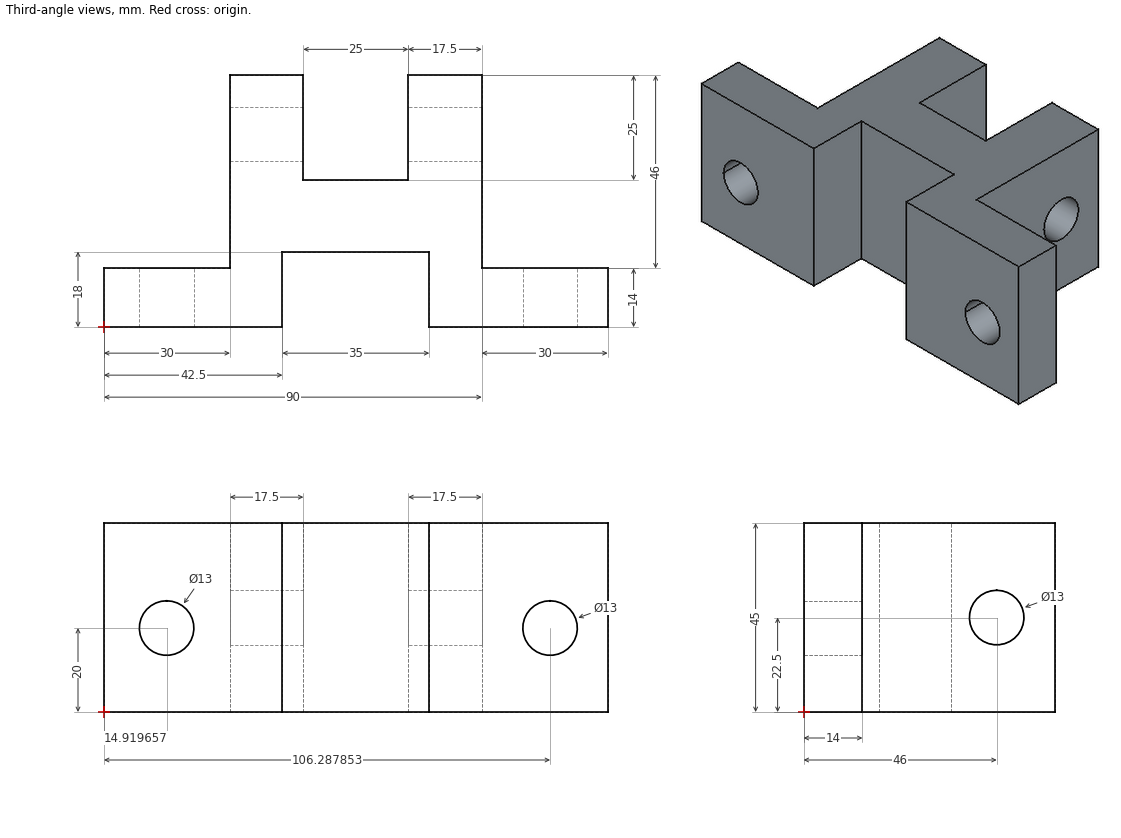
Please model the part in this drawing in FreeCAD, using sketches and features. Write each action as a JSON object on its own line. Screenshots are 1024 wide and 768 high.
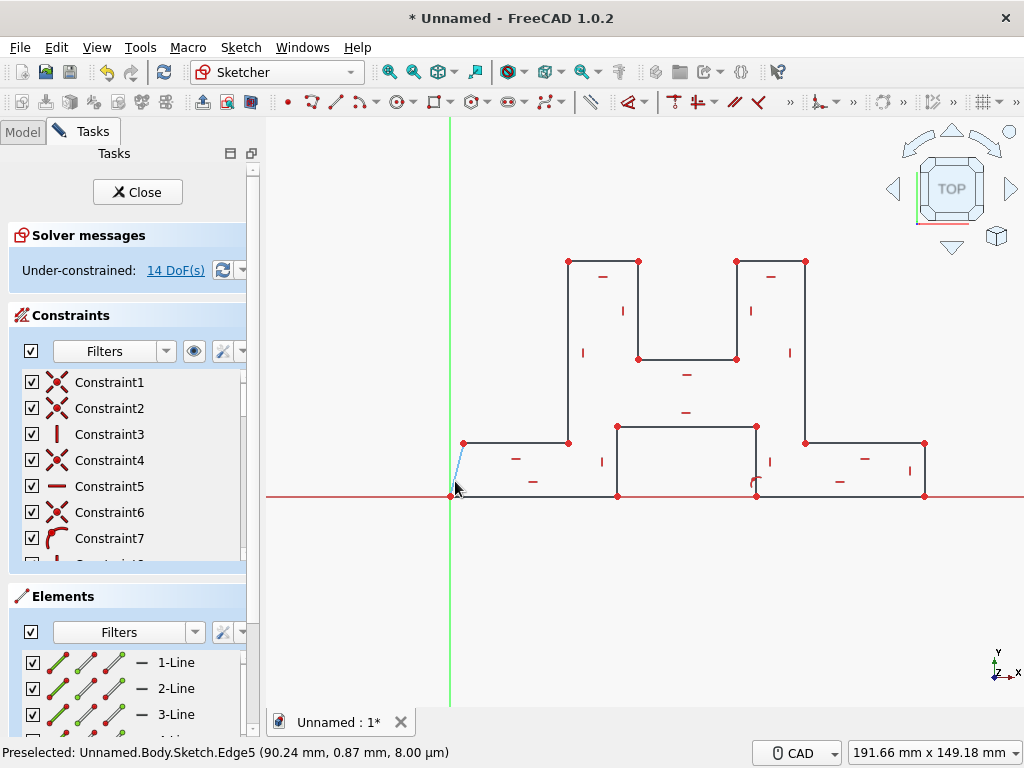
{"action": "left_click", "coordinate": [454, 481]}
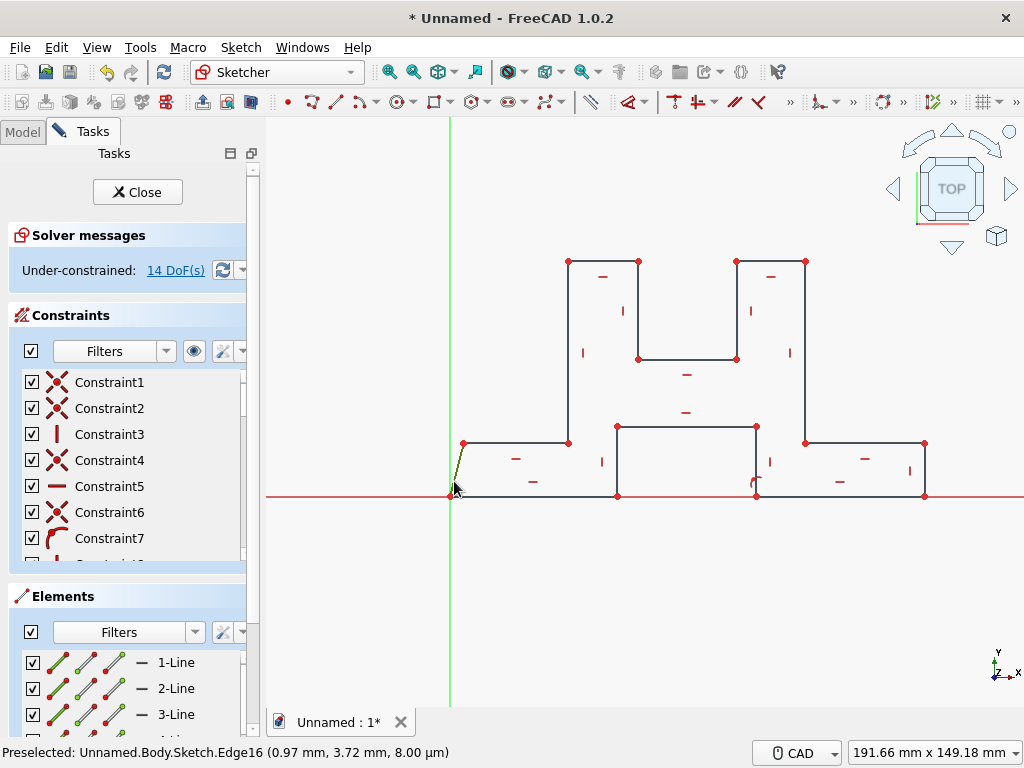
{"action": "left_click", "coordinate": [716, 102]}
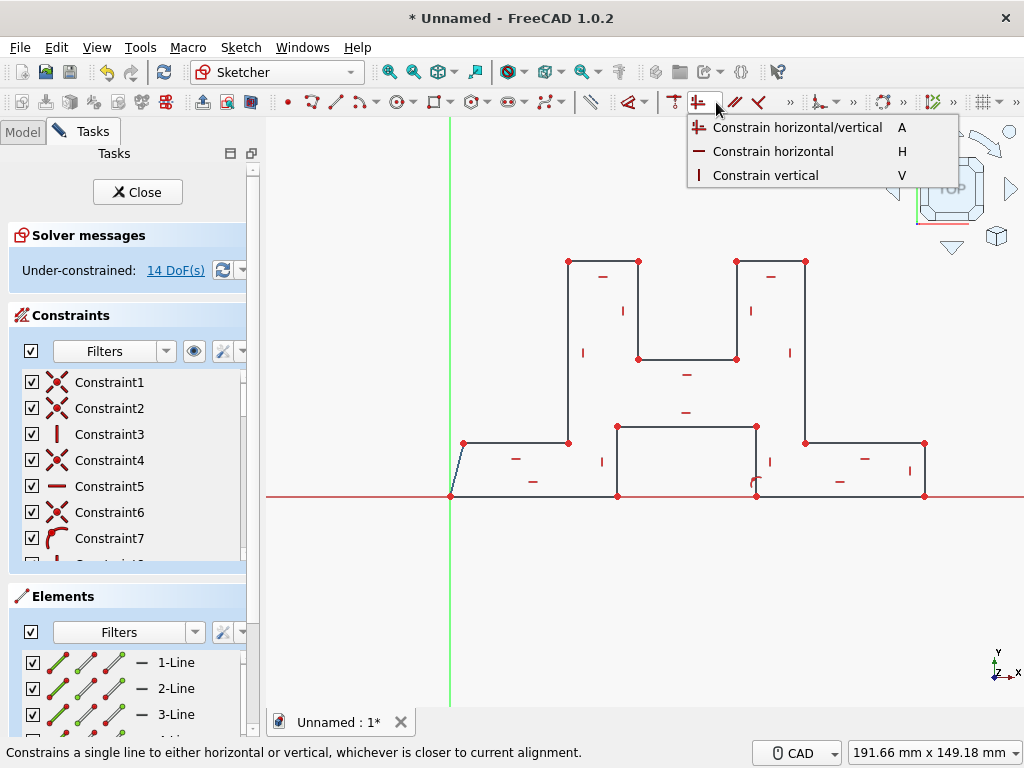
{"action": "left_click", "coordinate": [823, 175]}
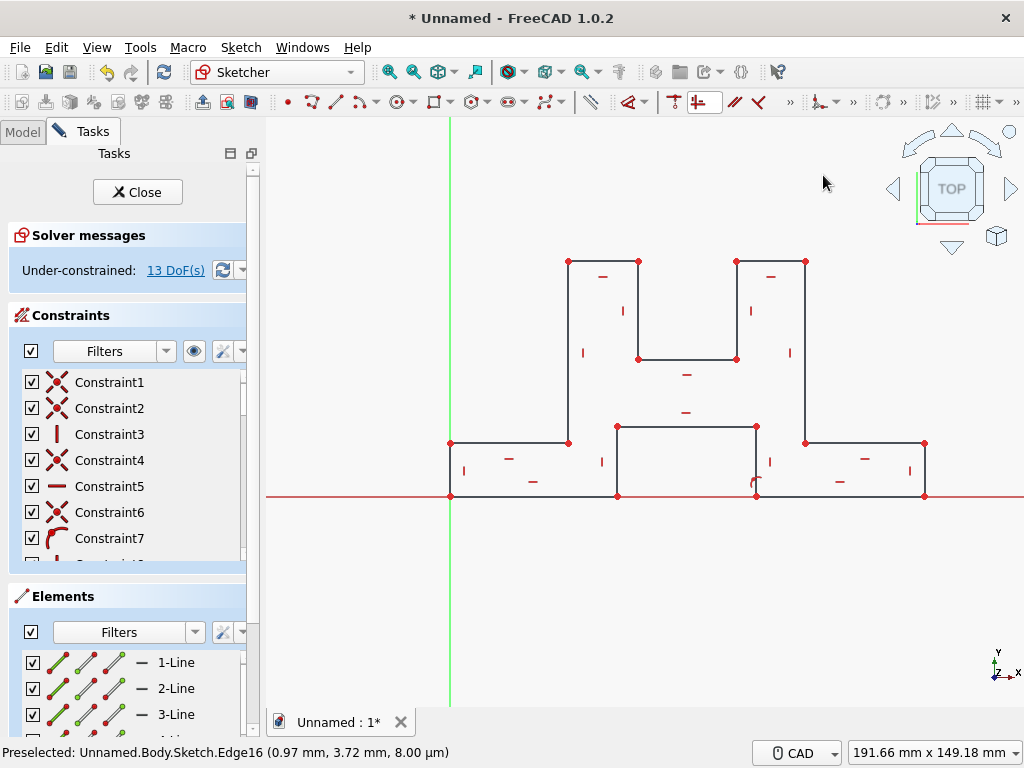
{"action": "left_click", "coordinate": [617, 476]}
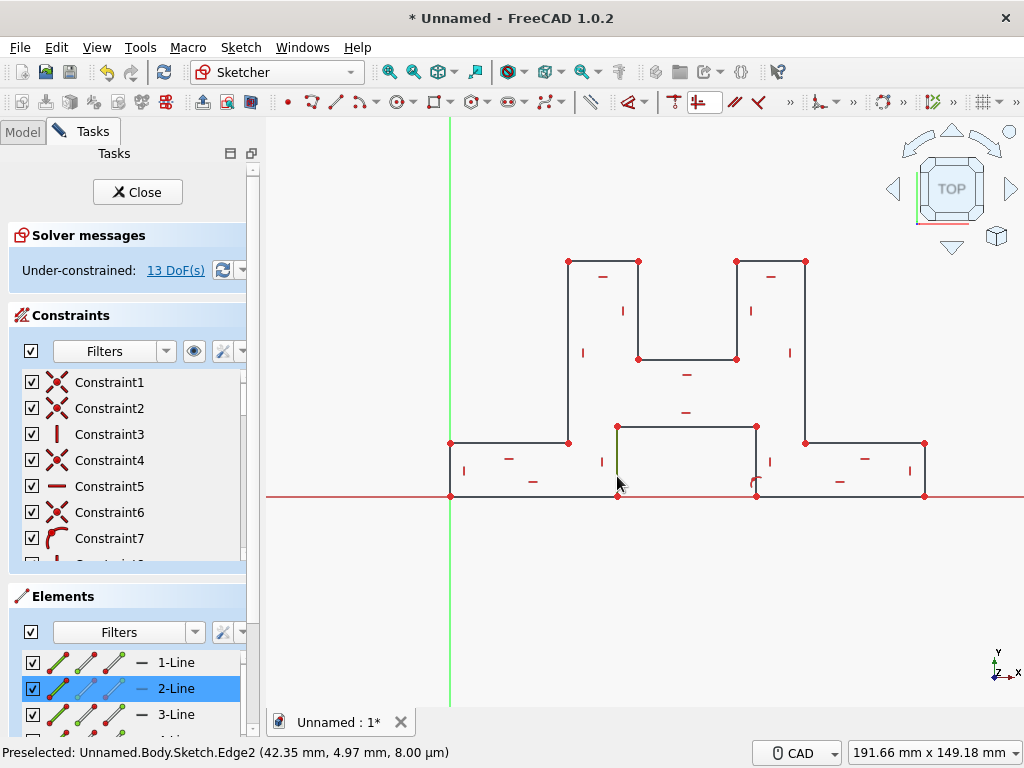
{"action": "key", "text": "i"}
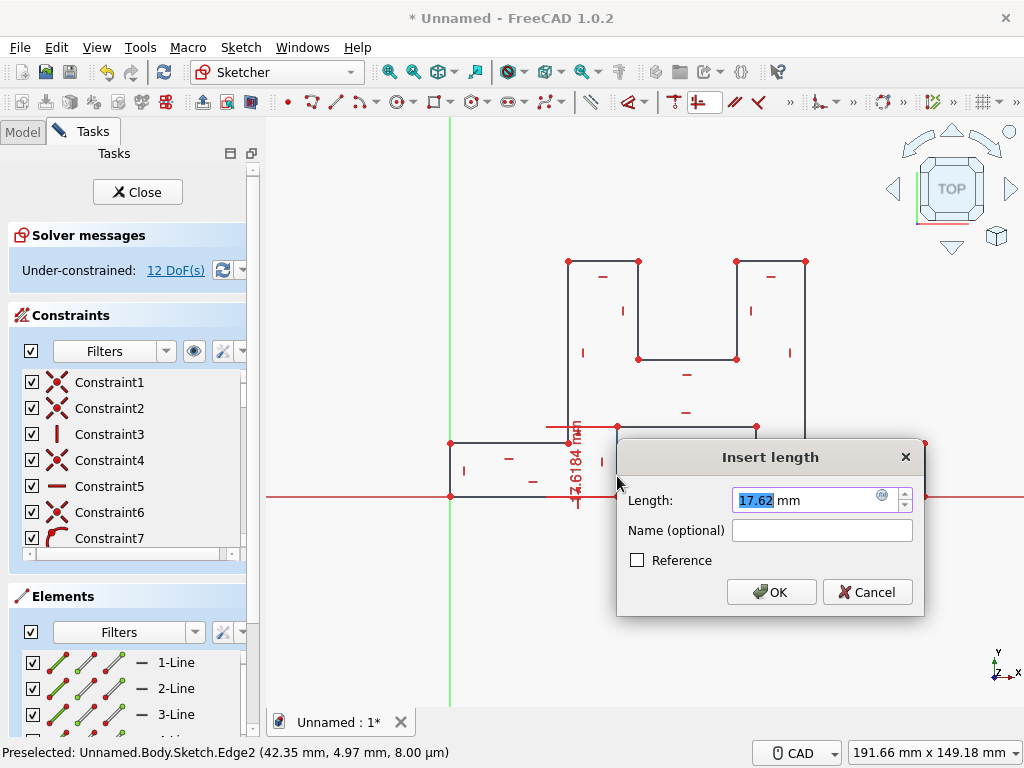
{"action": "type", "text": "18"}
{"action": "key", "text": "Return"}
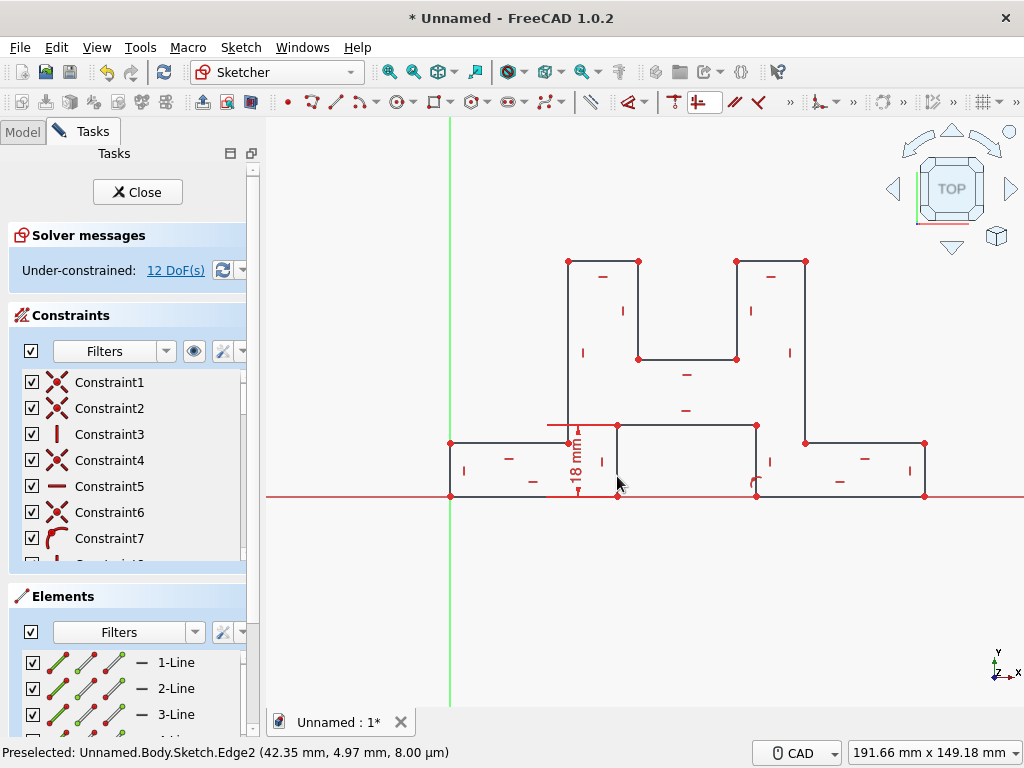
{"action": "left_click", "coordinate": [659, 425]}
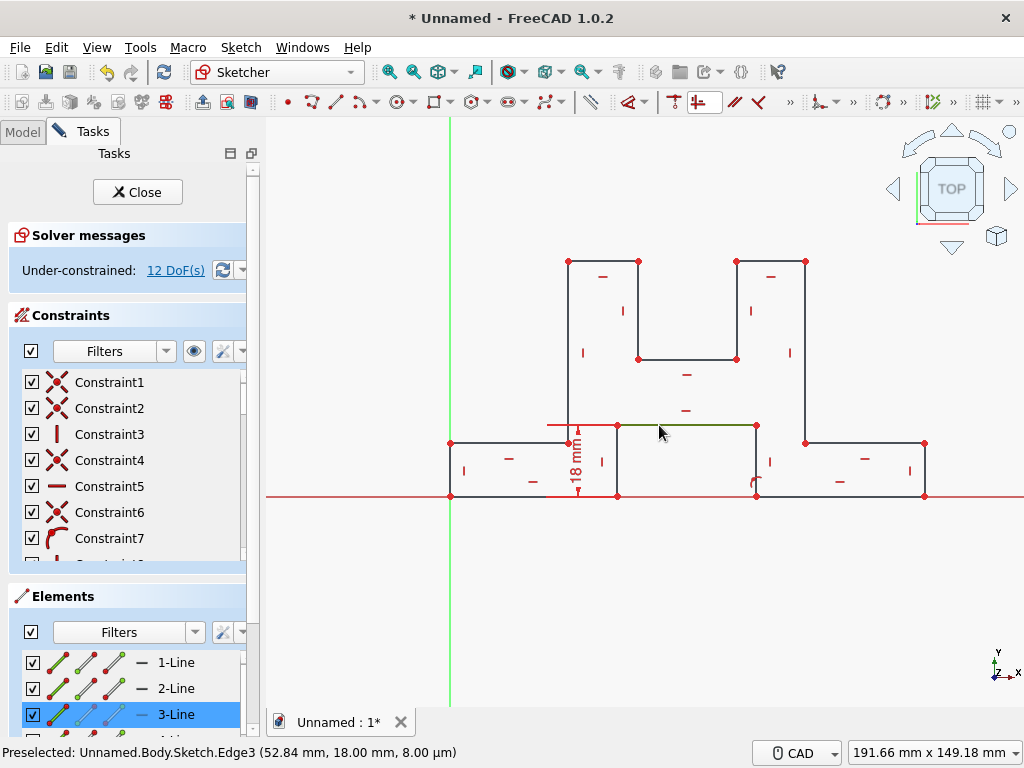
{"action": "key", "text": "l"}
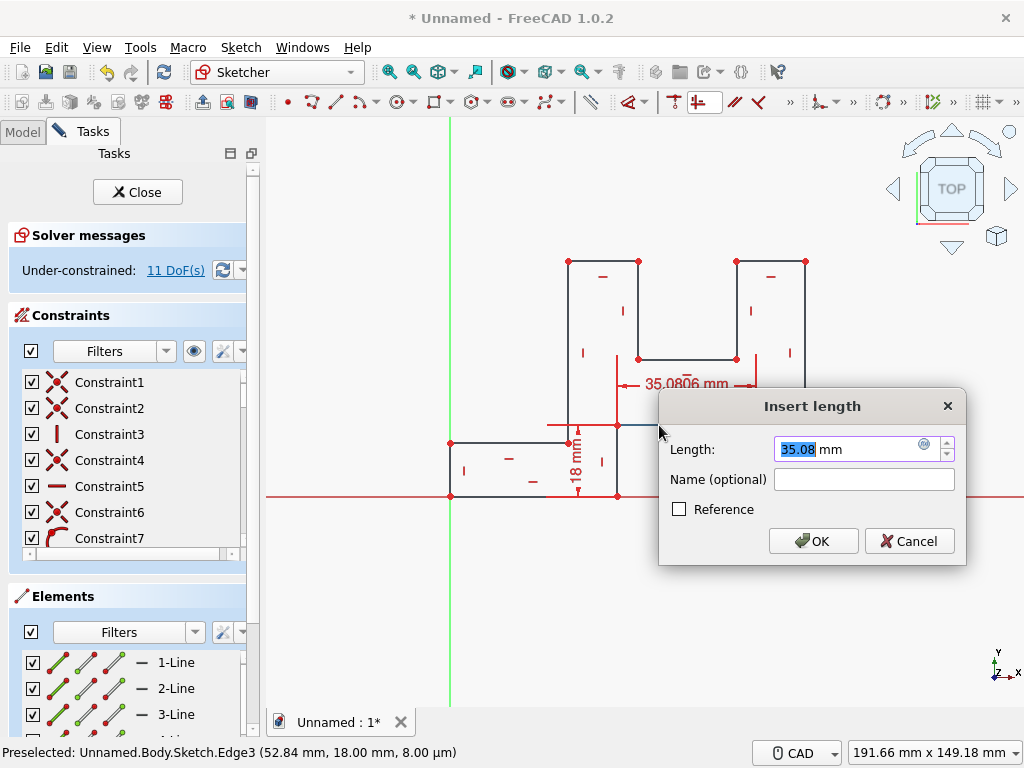
{"action": "type", "text": "35"}
{"action": "key", "text": "Return"}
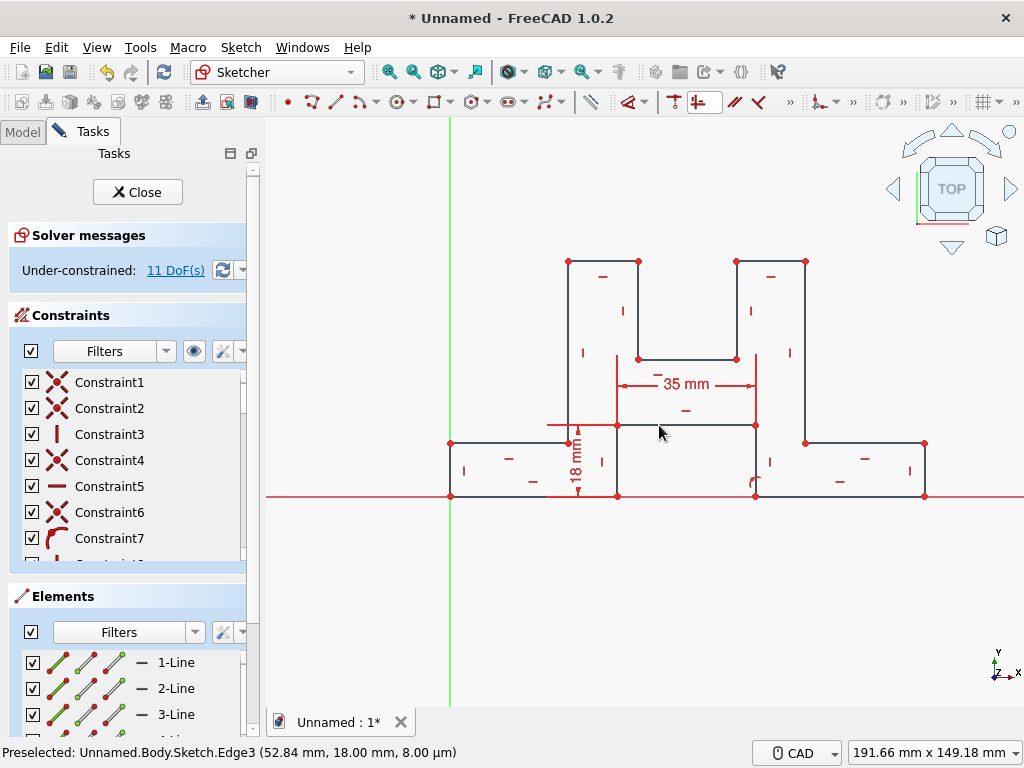
{"action": "scroll", "coordinate": [294, 565], "scroll_direction": "down", "scroll_amount": 1}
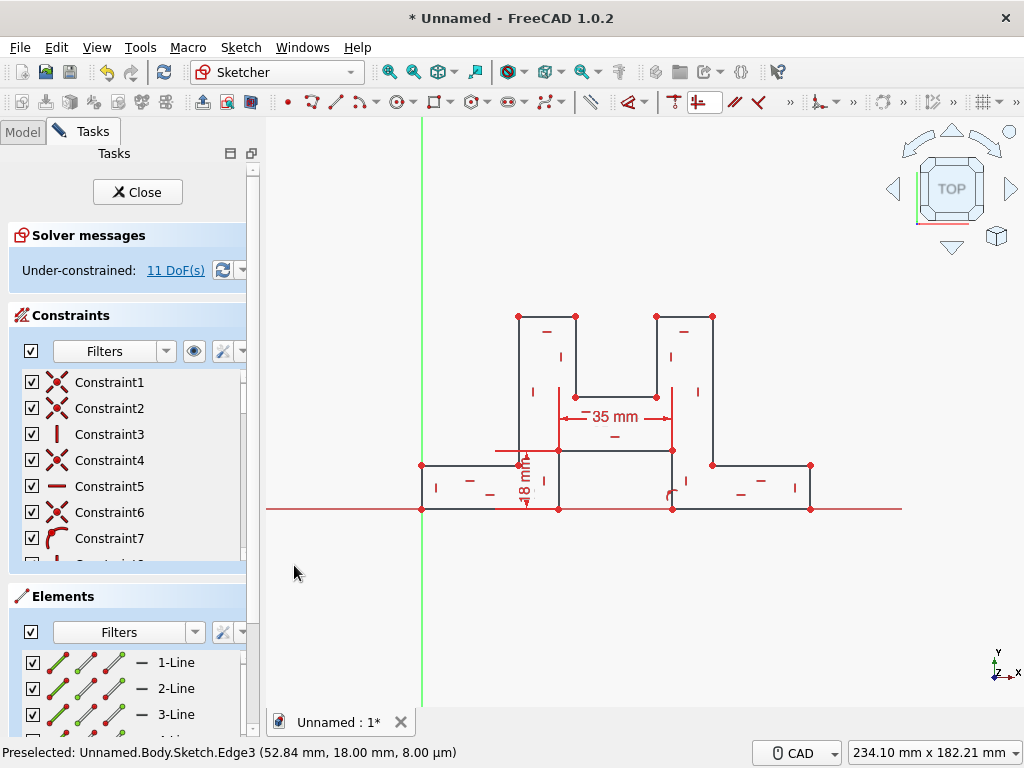
{"action": "left_click", "coordinate": [810, 496]}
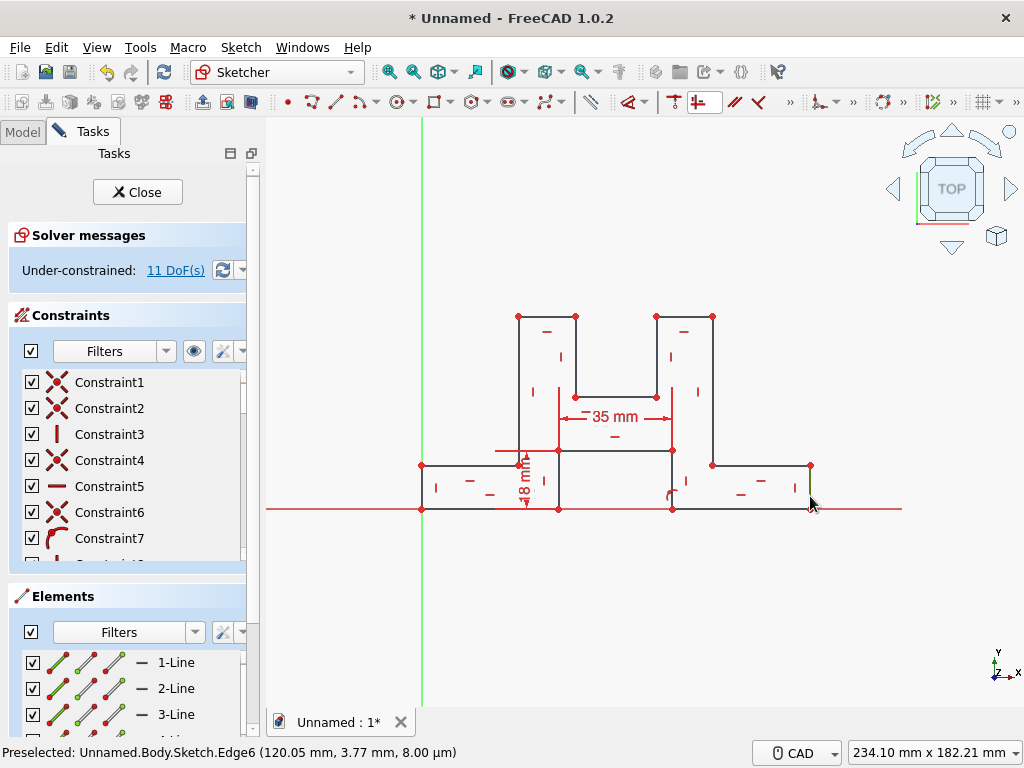
{"action": "key", "text": "i"}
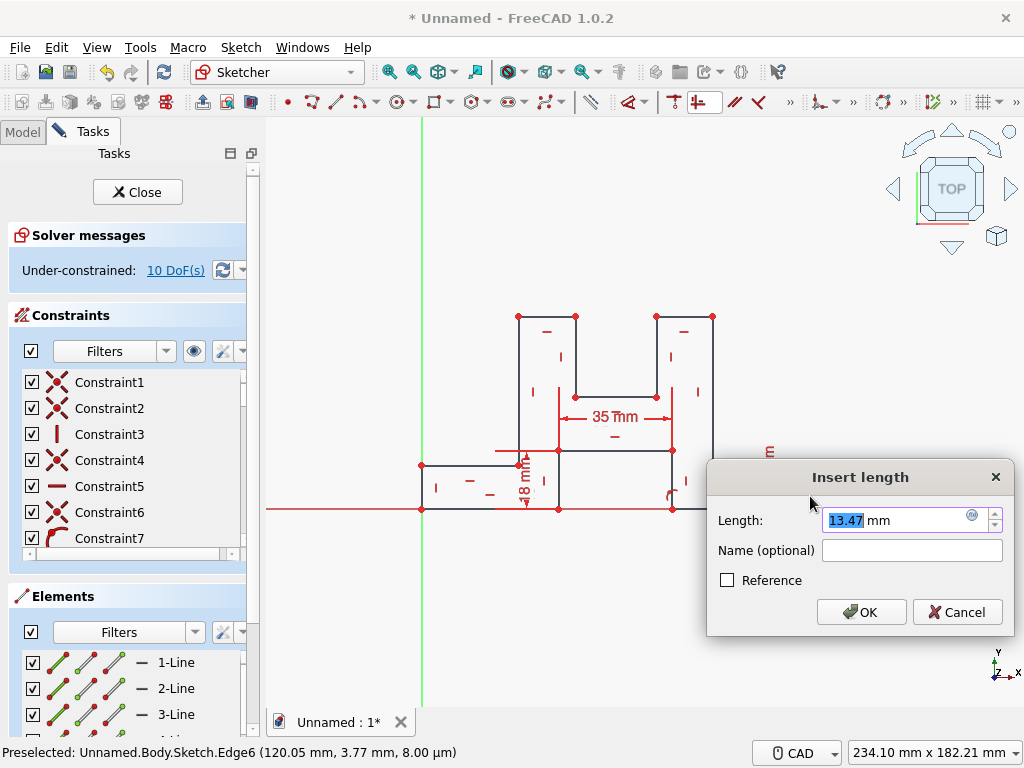
{"action": "type", "text": "14"}
{"action": "key", "text": "Return"}